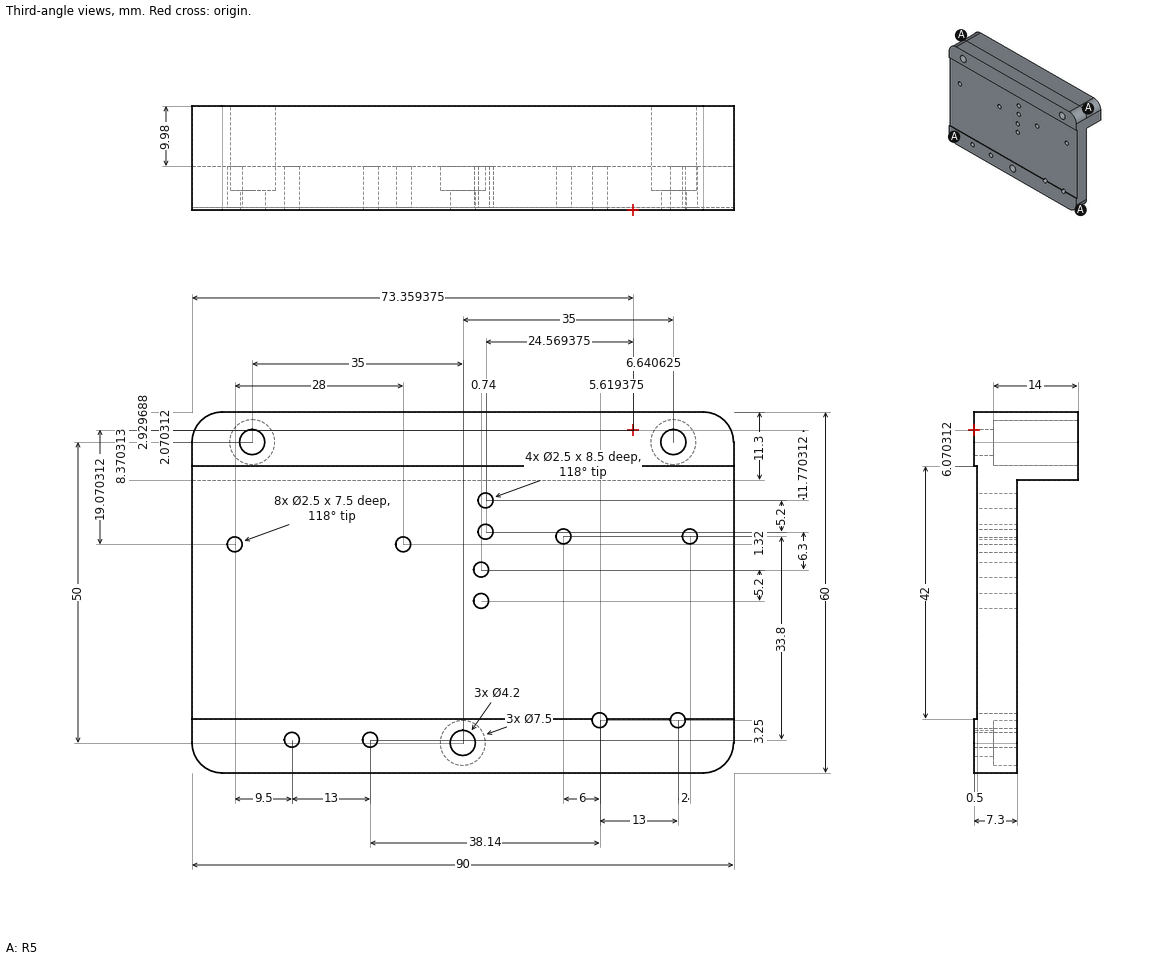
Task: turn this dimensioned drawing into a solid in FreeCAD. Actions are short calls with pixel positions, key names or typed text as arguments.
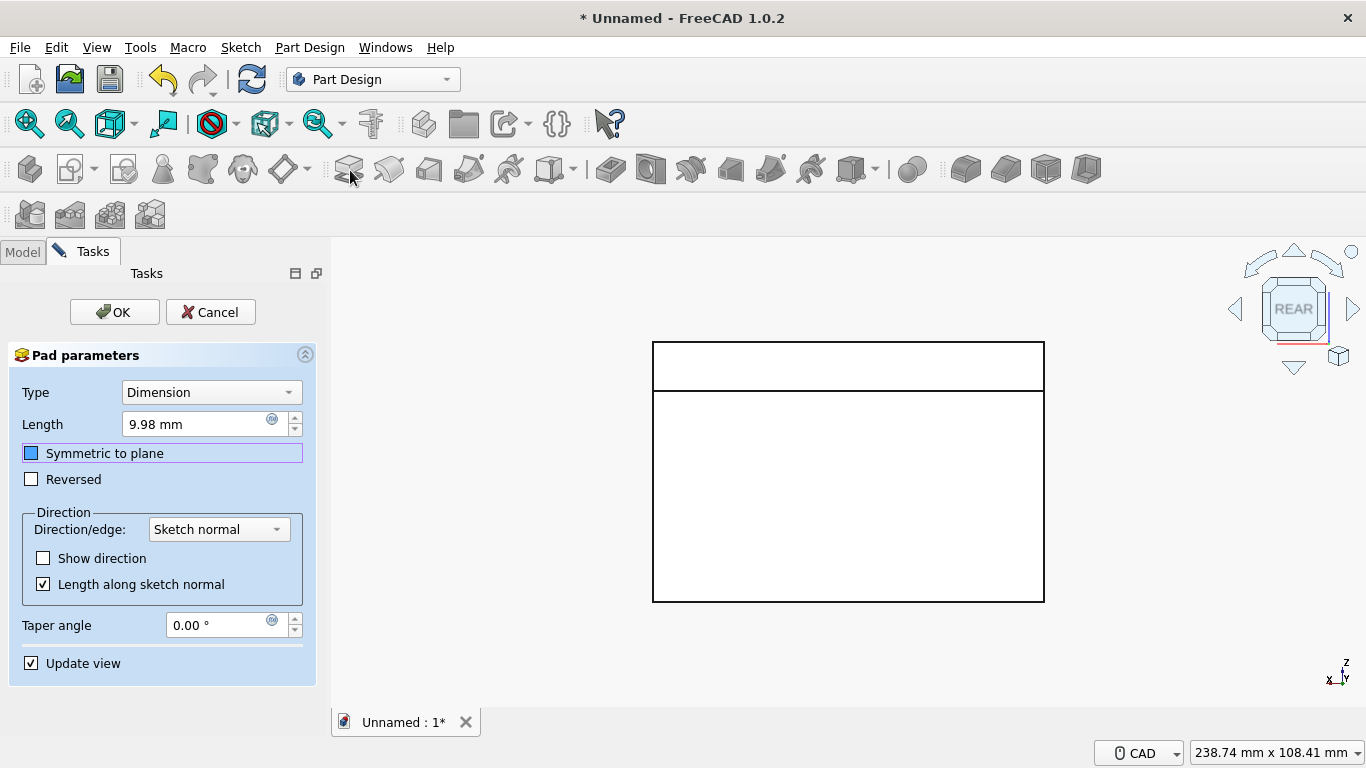
click(115, 312)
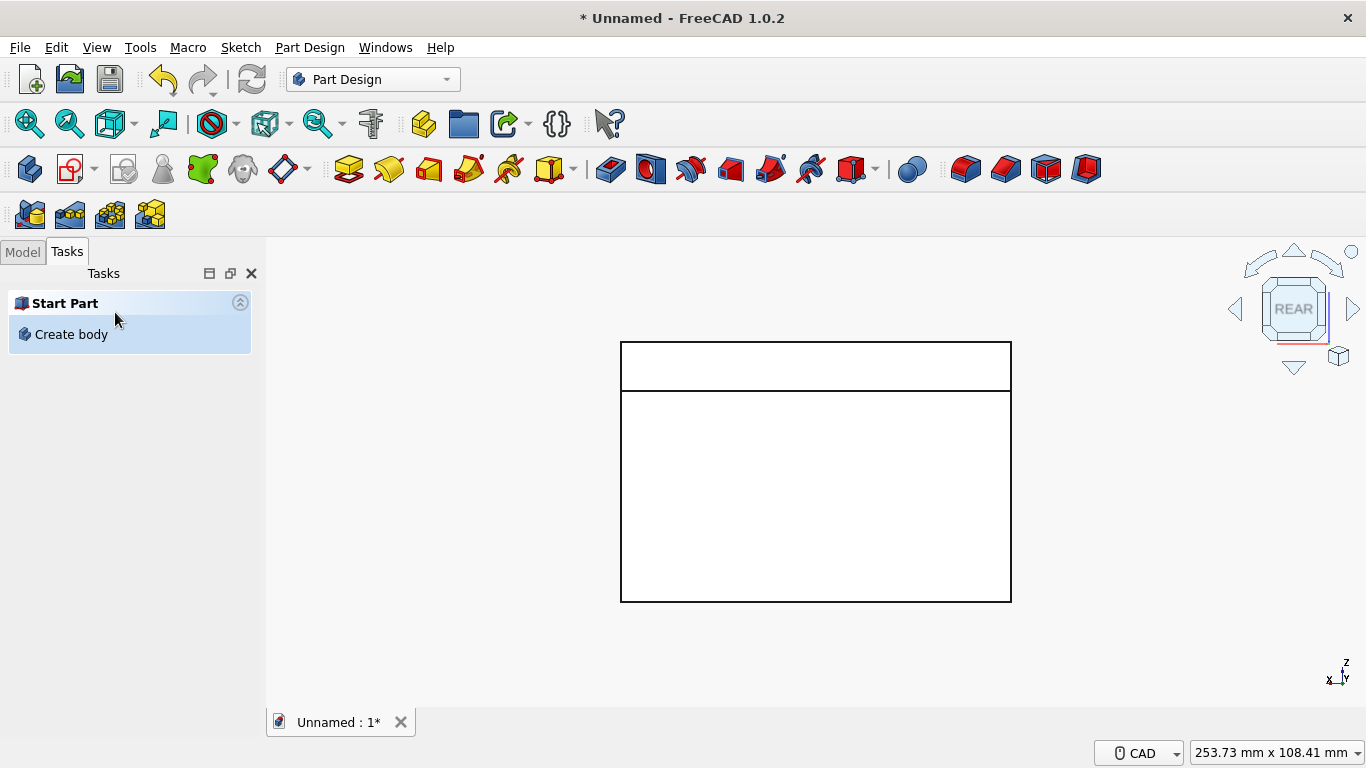
click(760, 495)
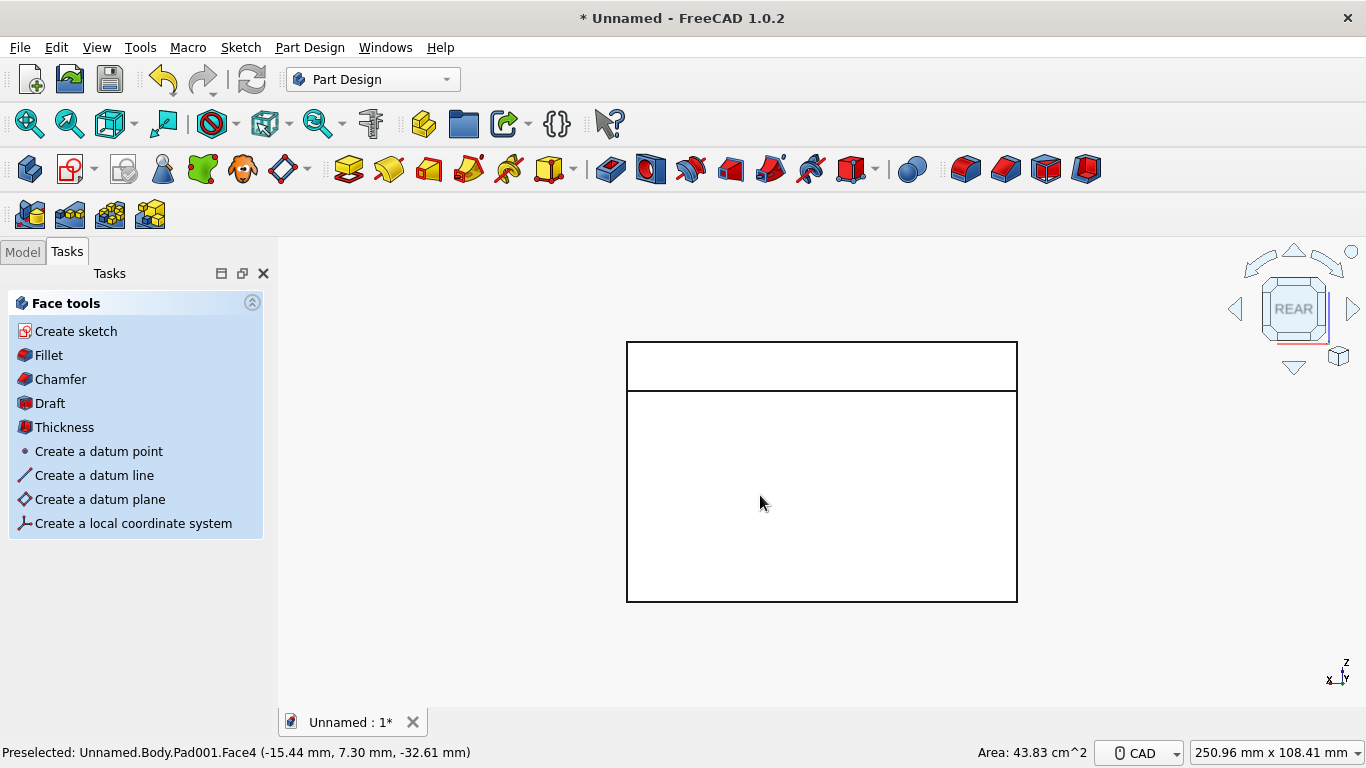
click(70, 170)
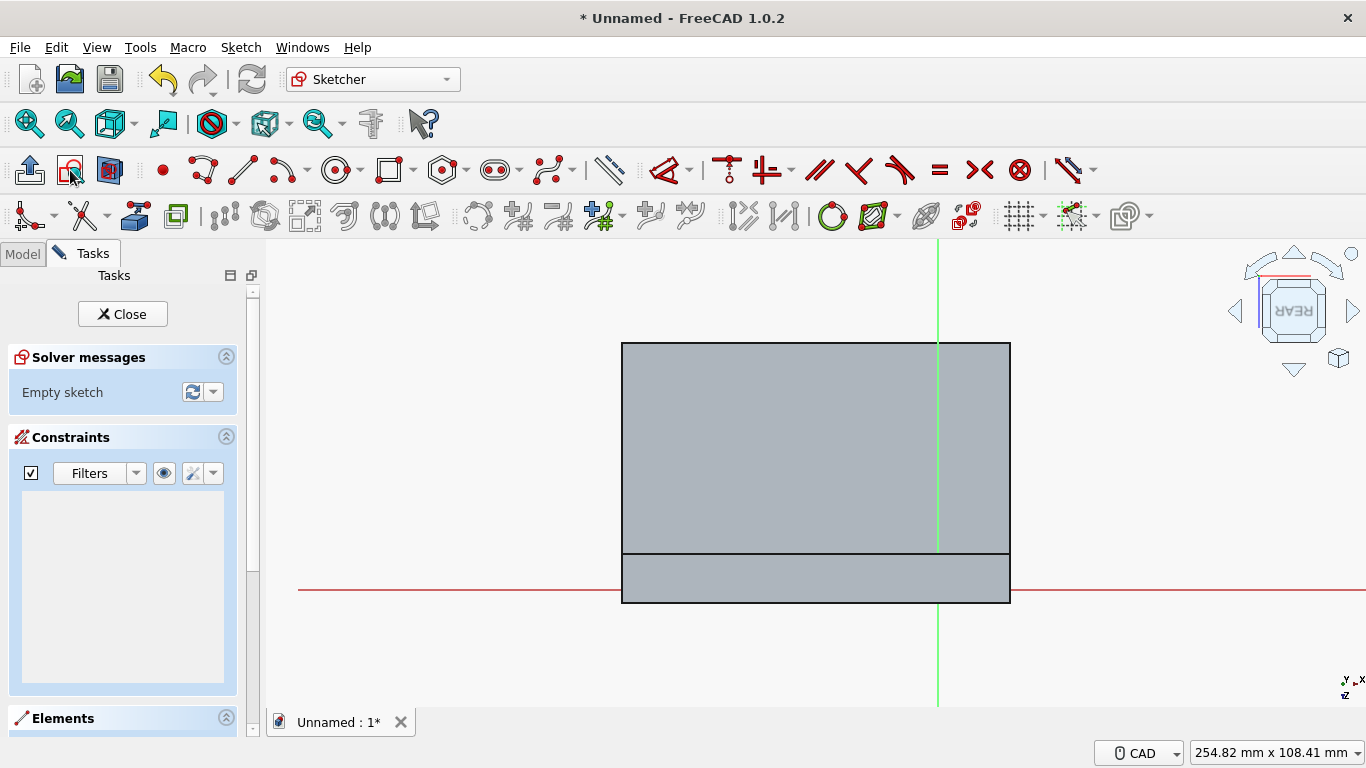
click(336, 170)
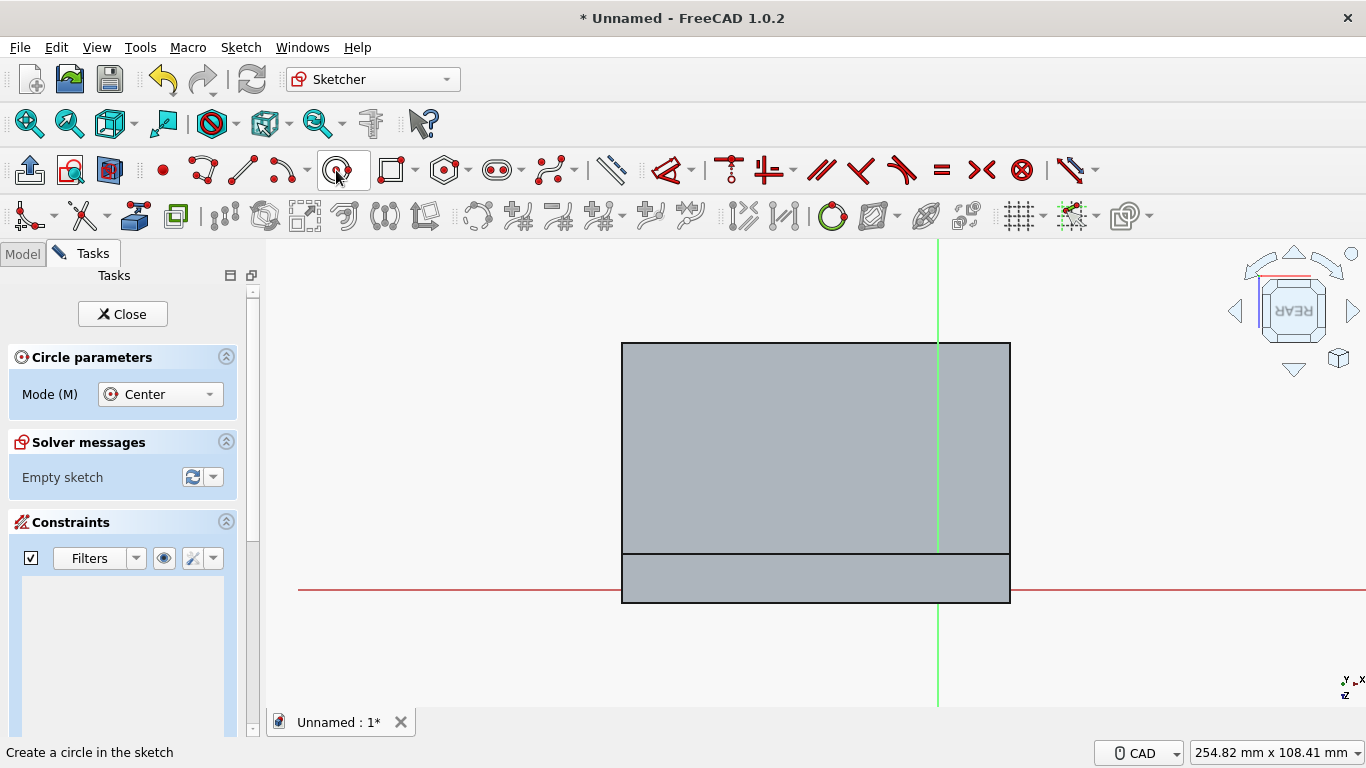
scroll(652, 508, up, 8)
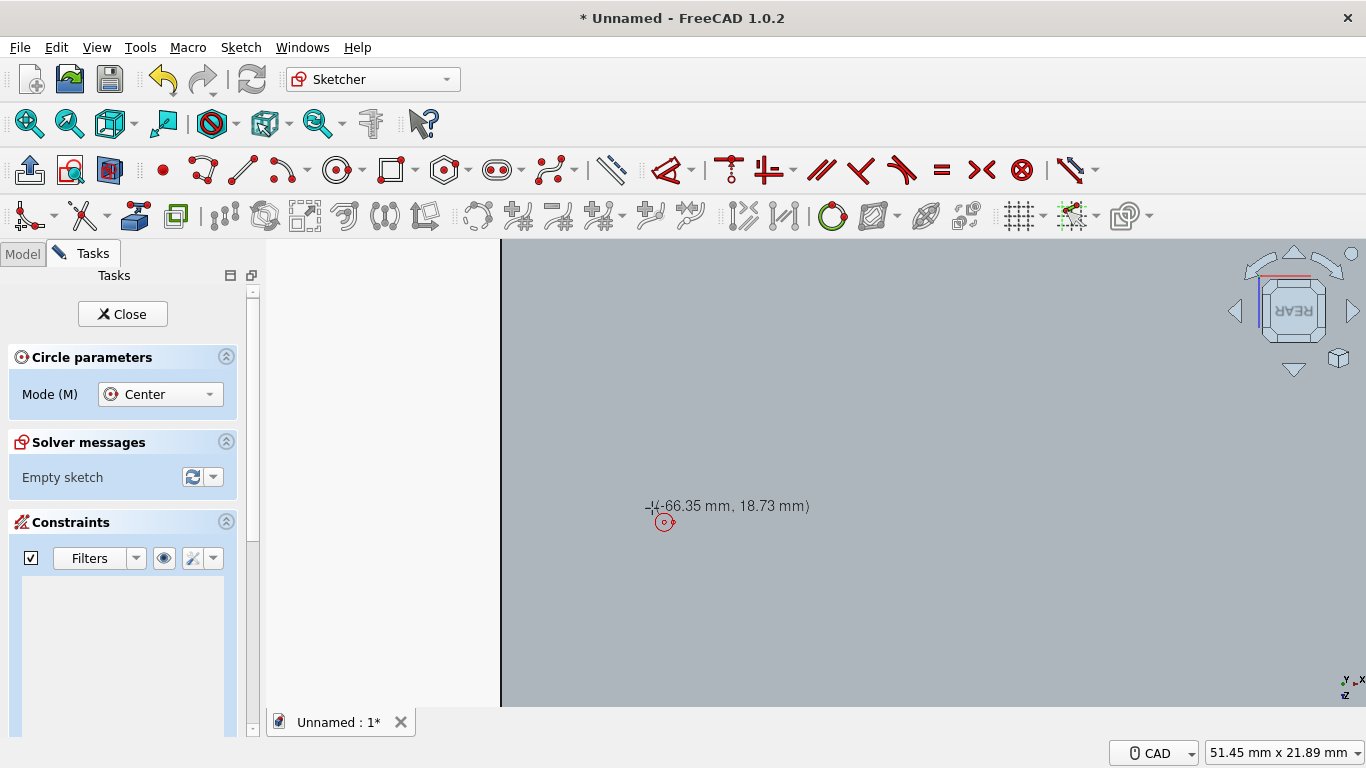
scroll(514, 514, down, 7)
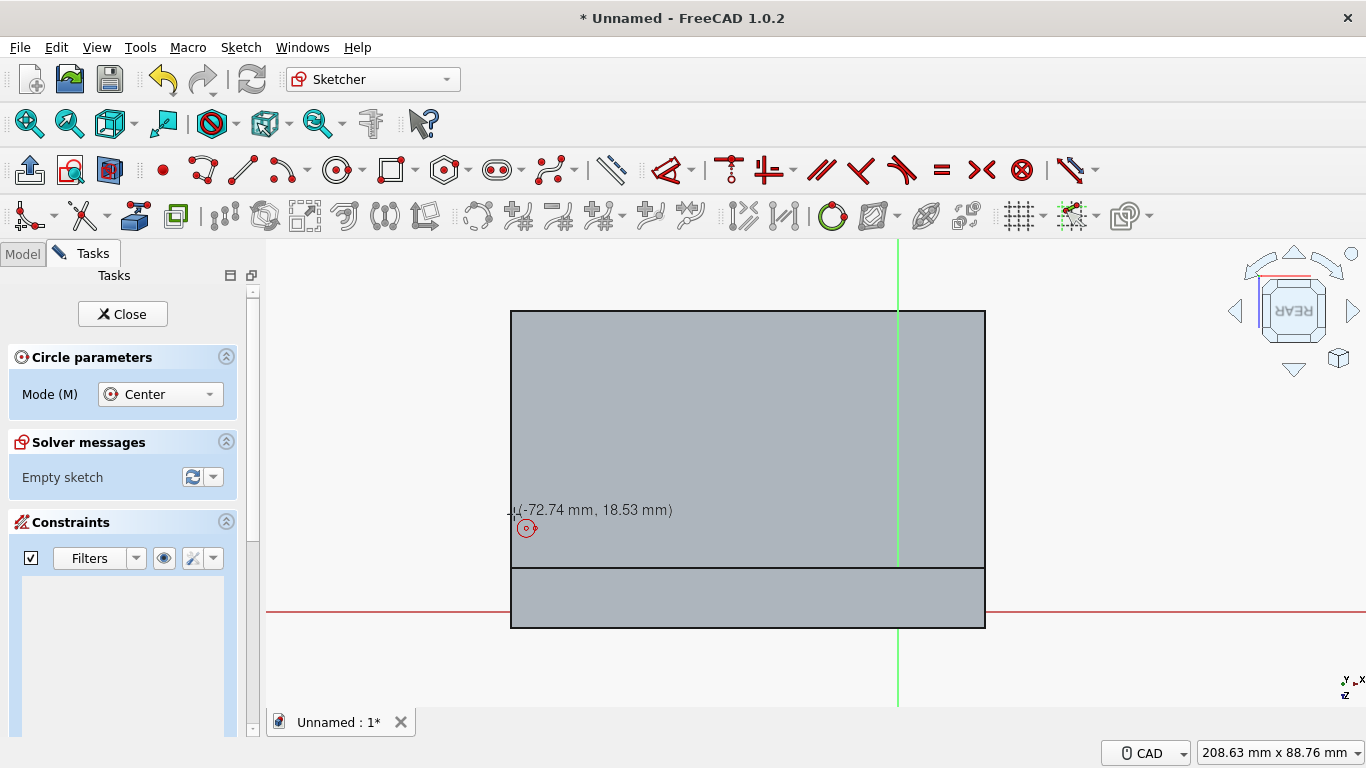
click(548, 512)
move(553, 507)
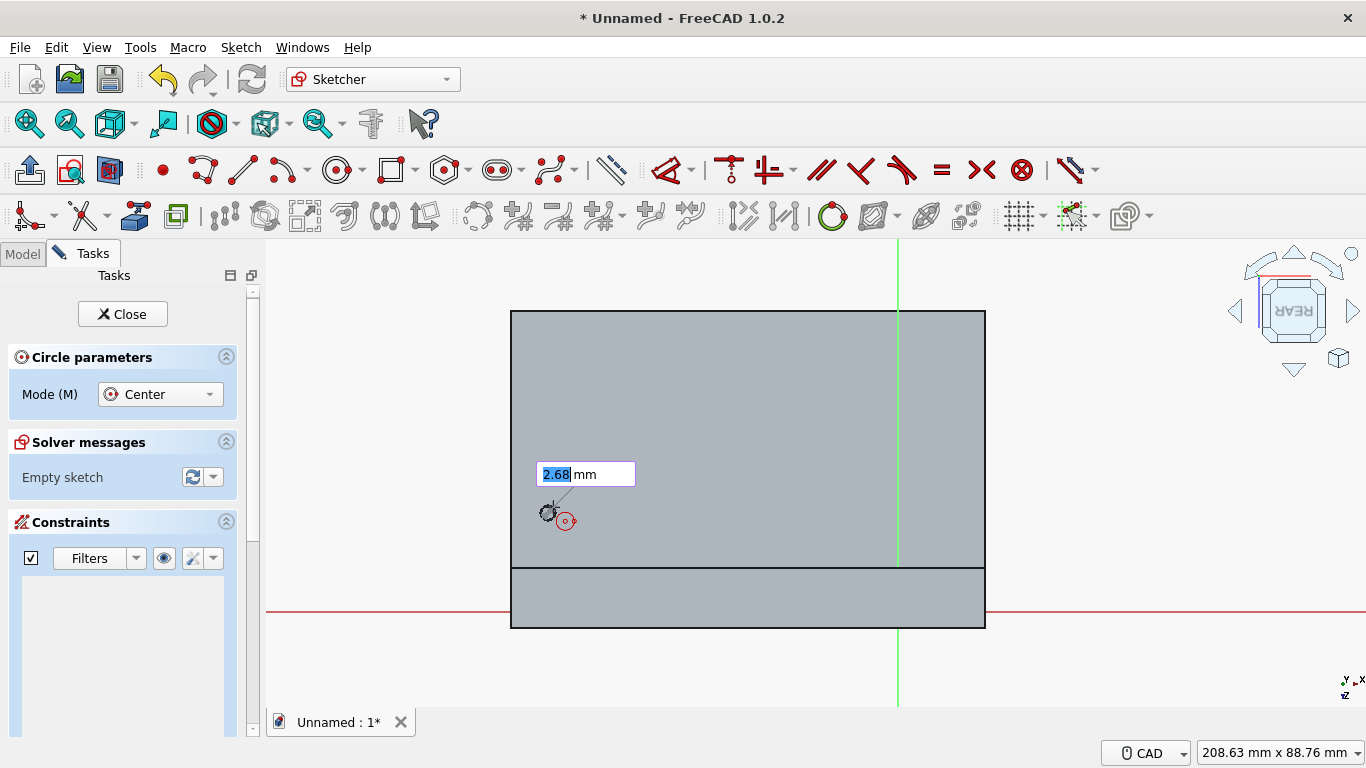
text(2.5)
key(Return)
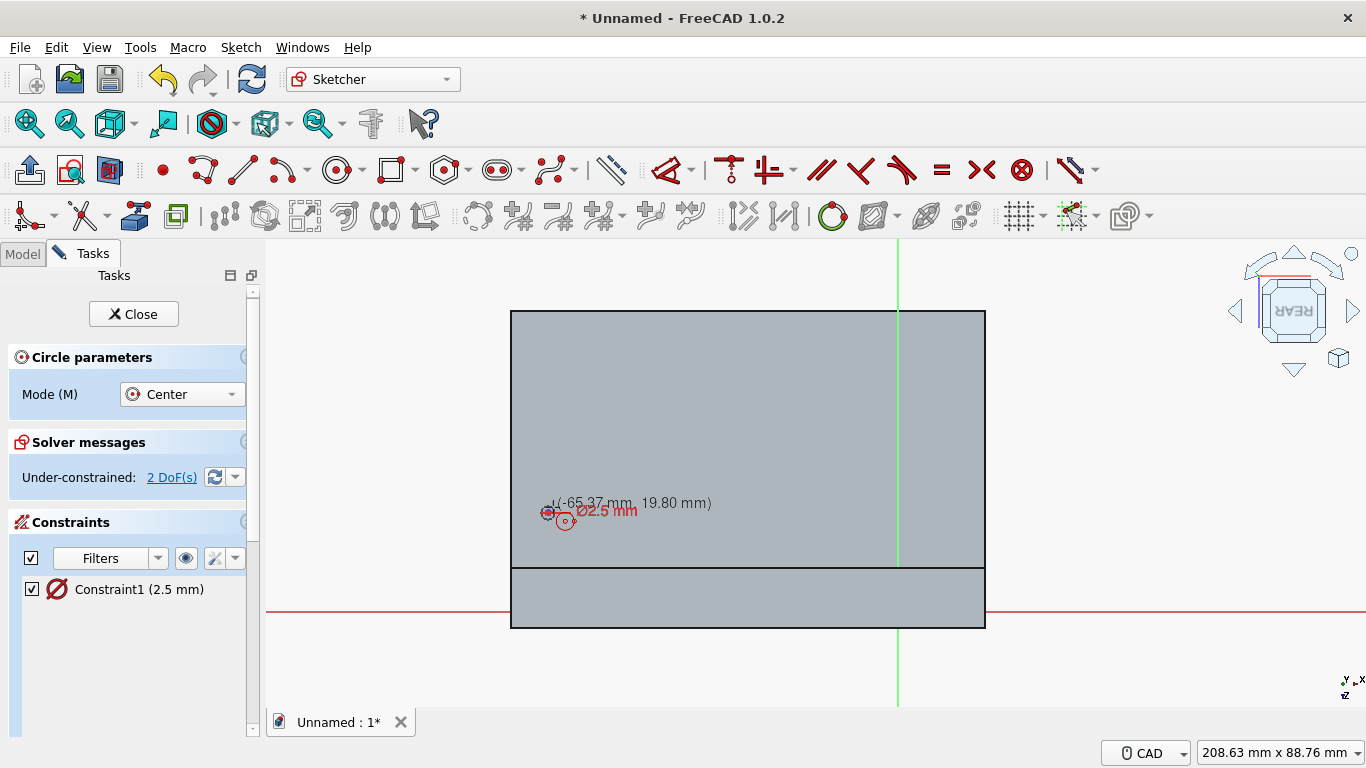
scroll(696, 512, up, 7)